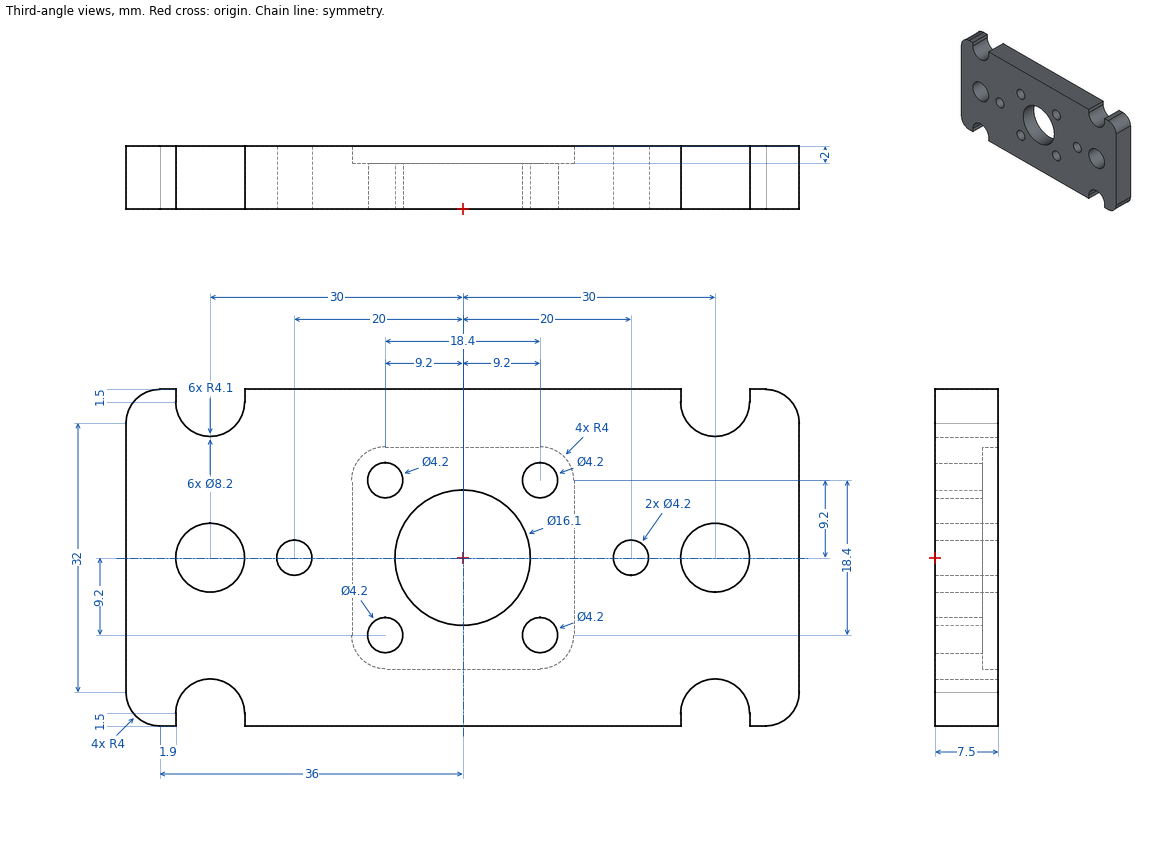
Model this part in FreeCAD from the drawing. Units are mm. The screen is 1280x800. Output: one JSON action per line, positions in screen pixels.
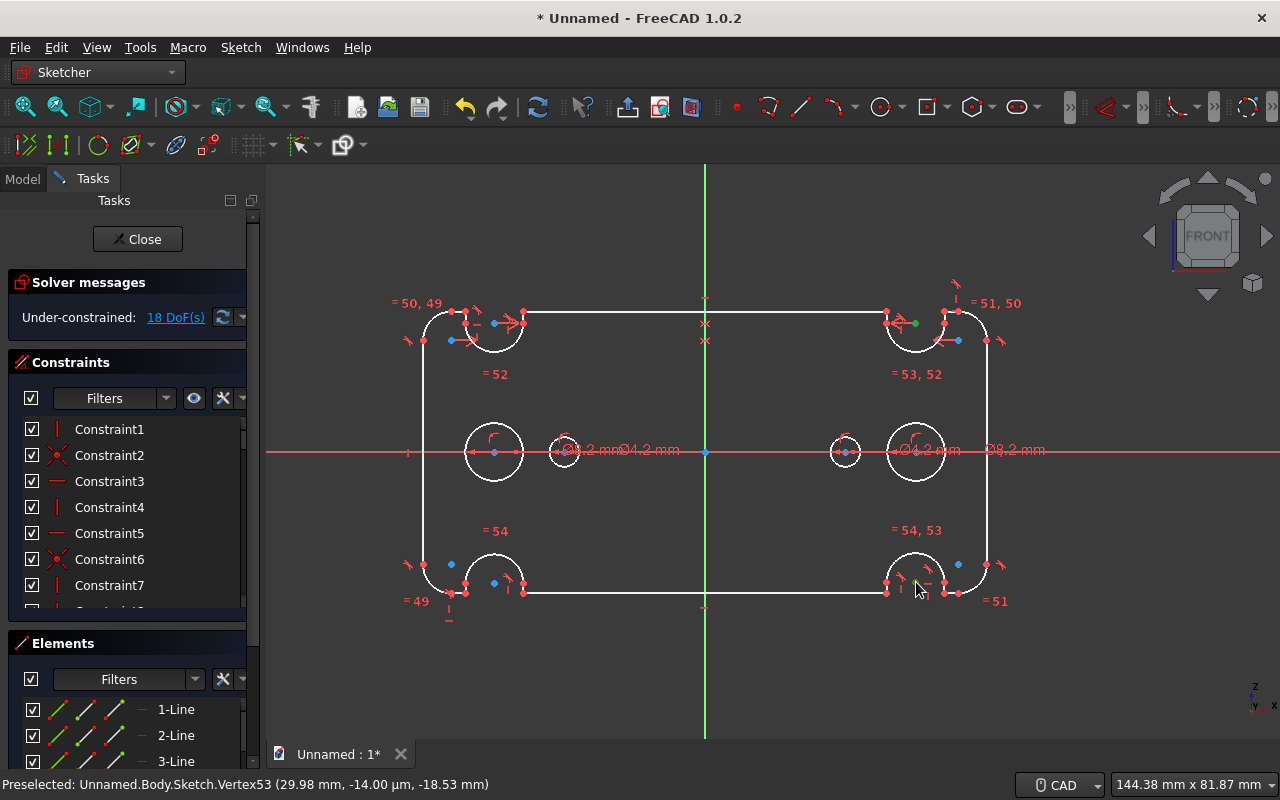
{"action": "left_click", "coordinate": [353, 452]}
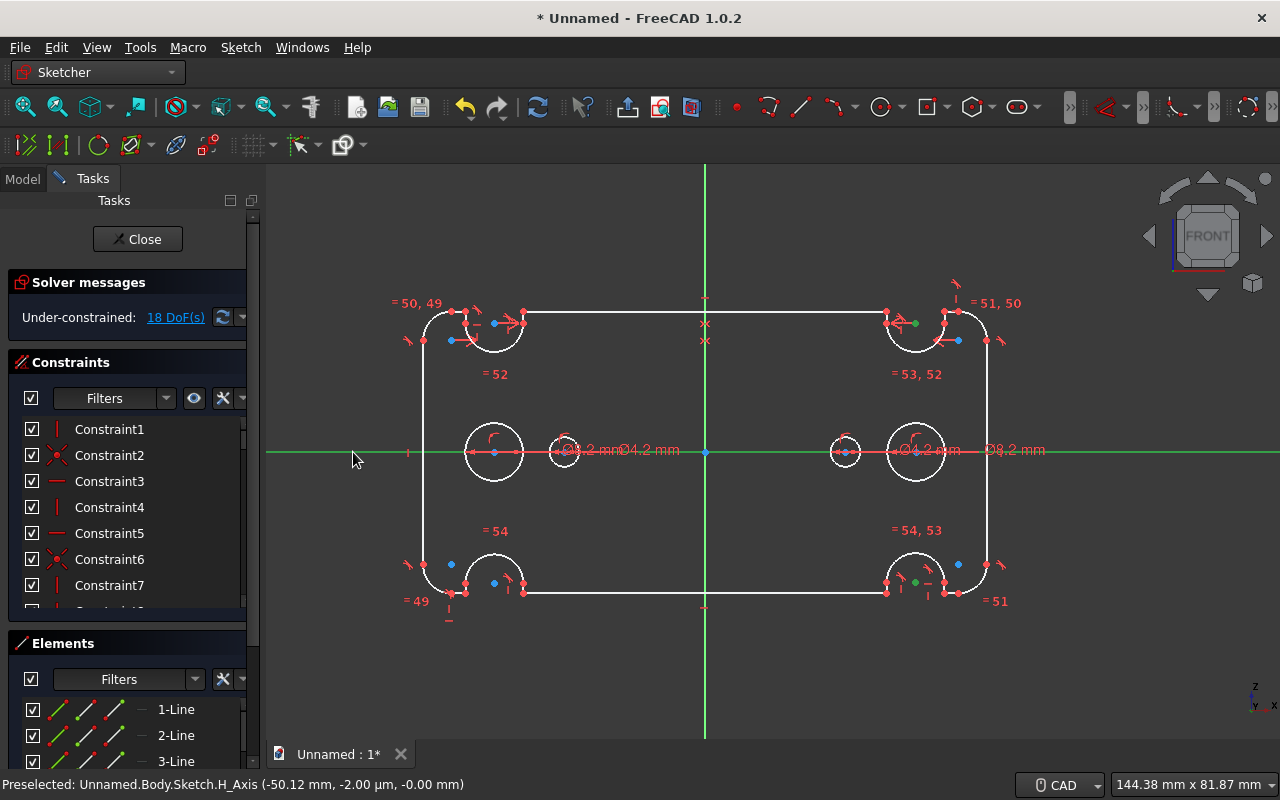
{"action": "key", "text": "s"}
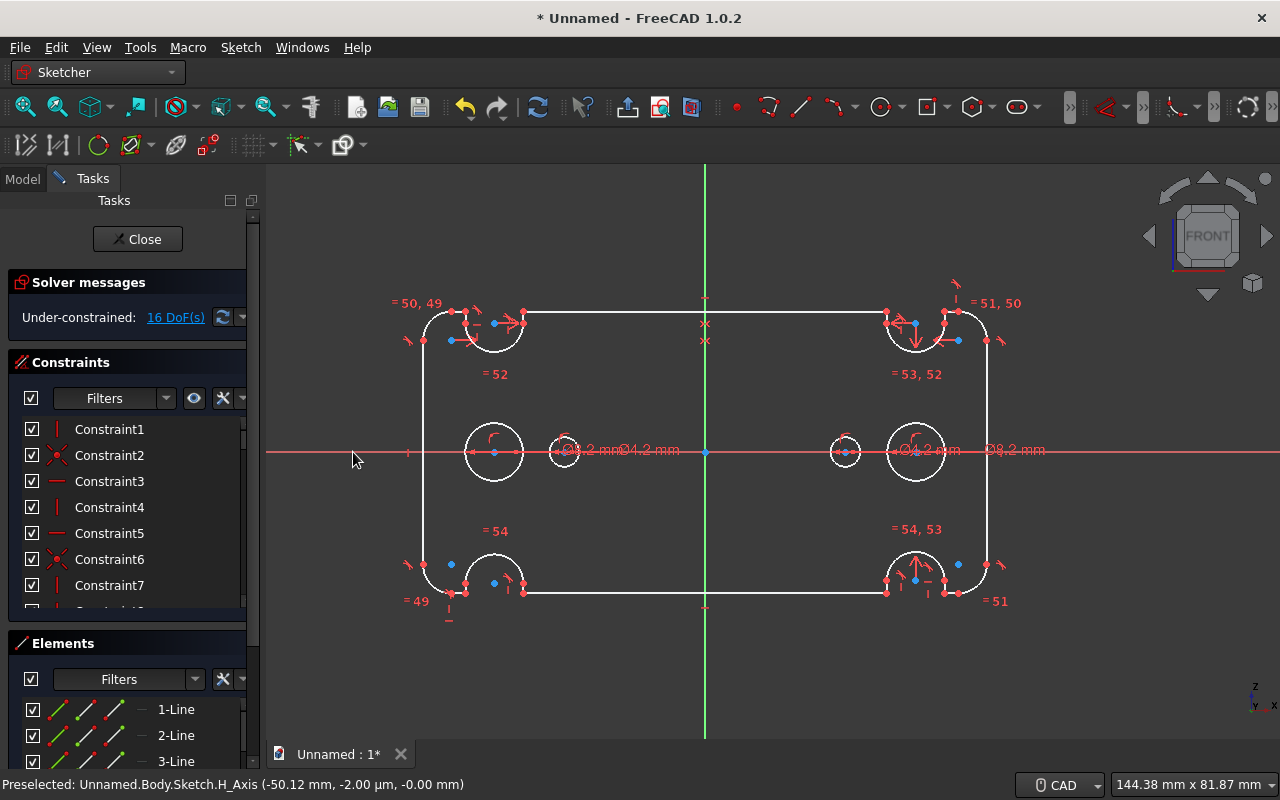
{"action": "left_click", "coordinate": [494, 323]}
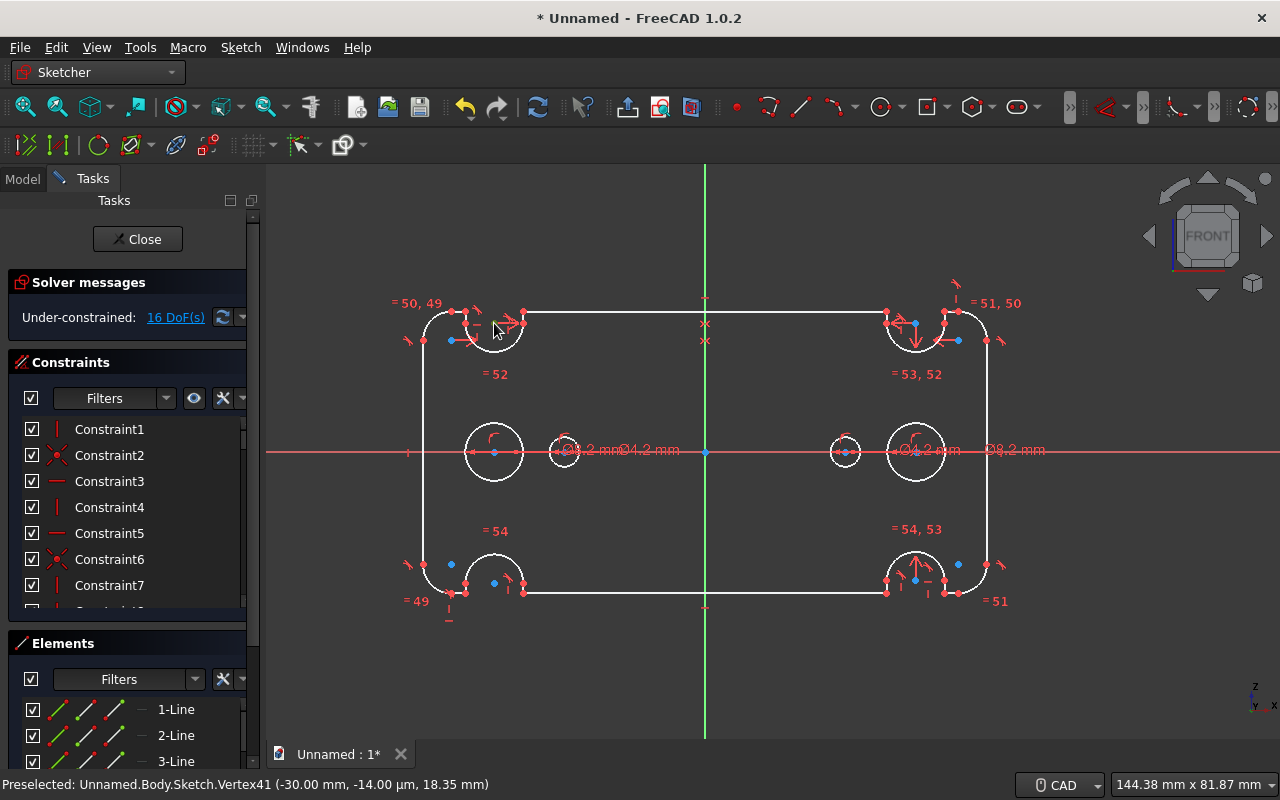
{"action": "left_click", "coordinate": [494, 583]}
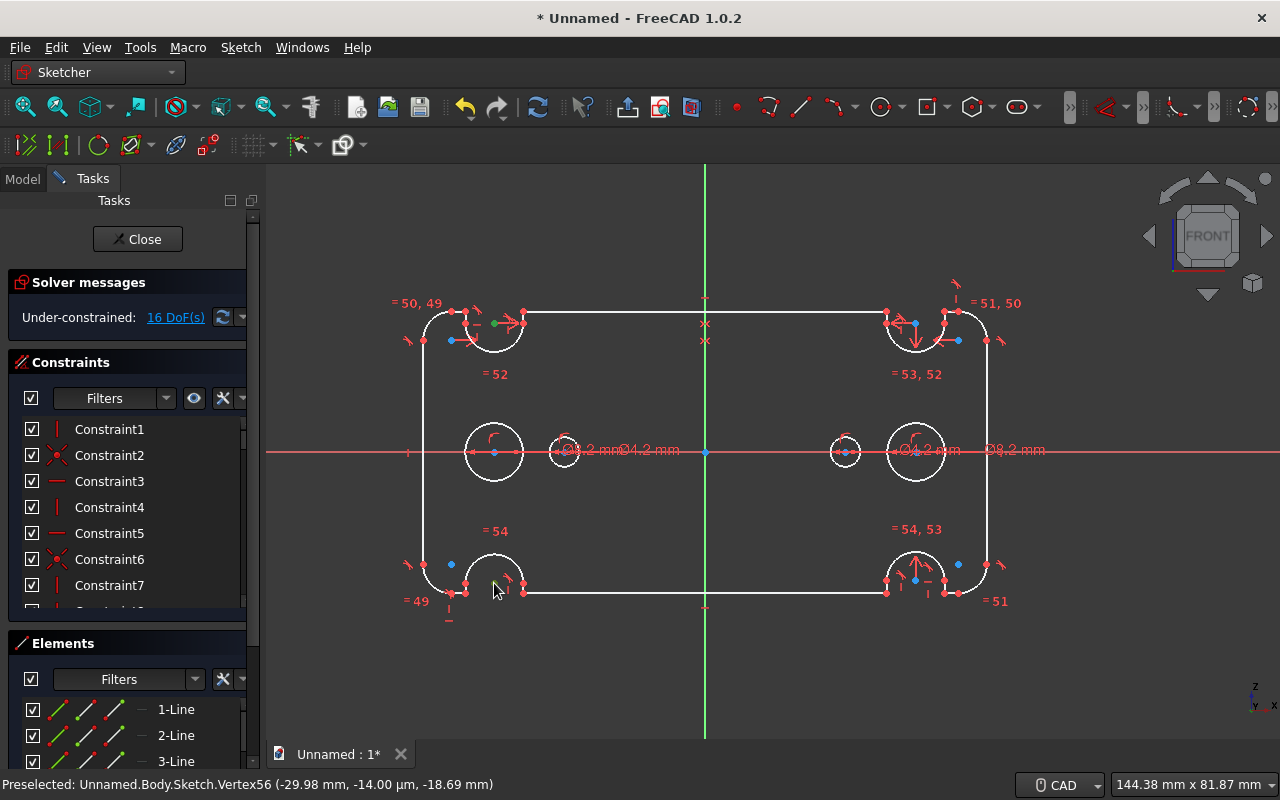
{"action": "left_click", "coordinate": [353, 452]}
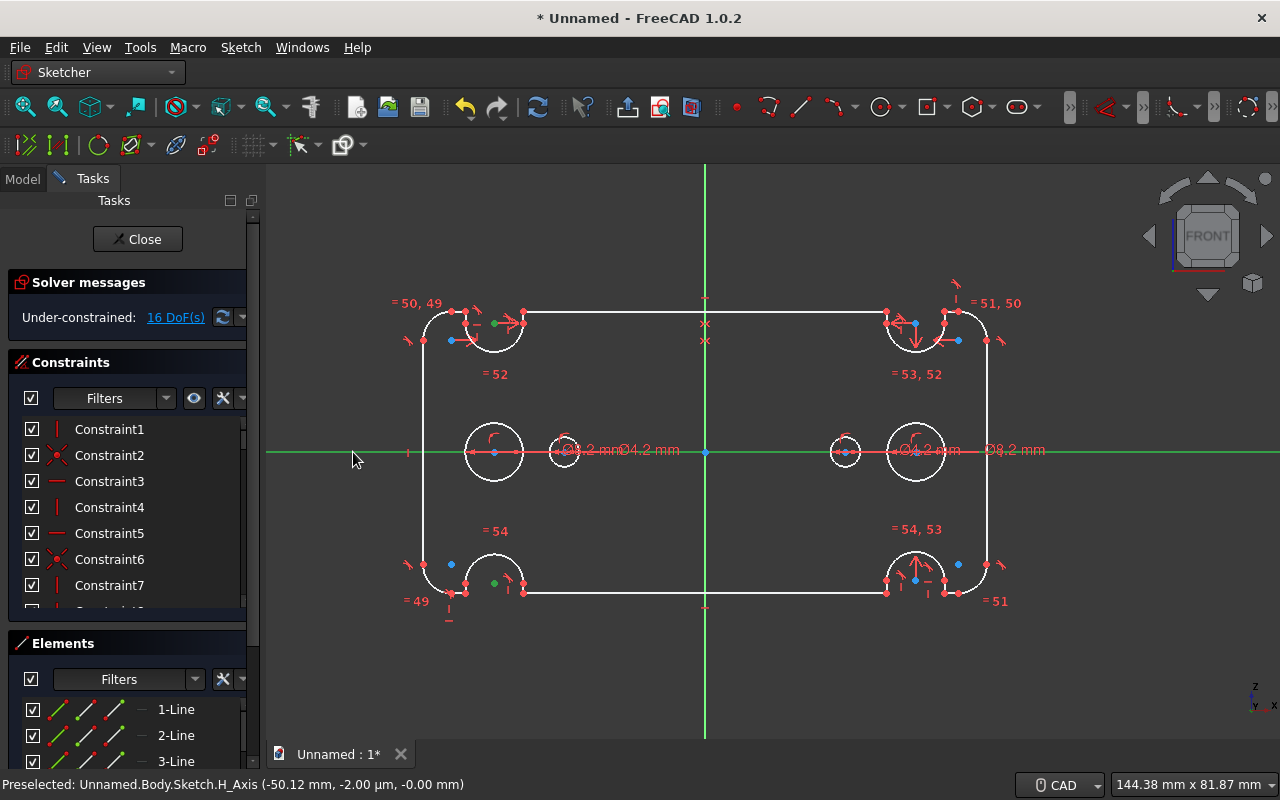
{"action": "key", "text": "s"}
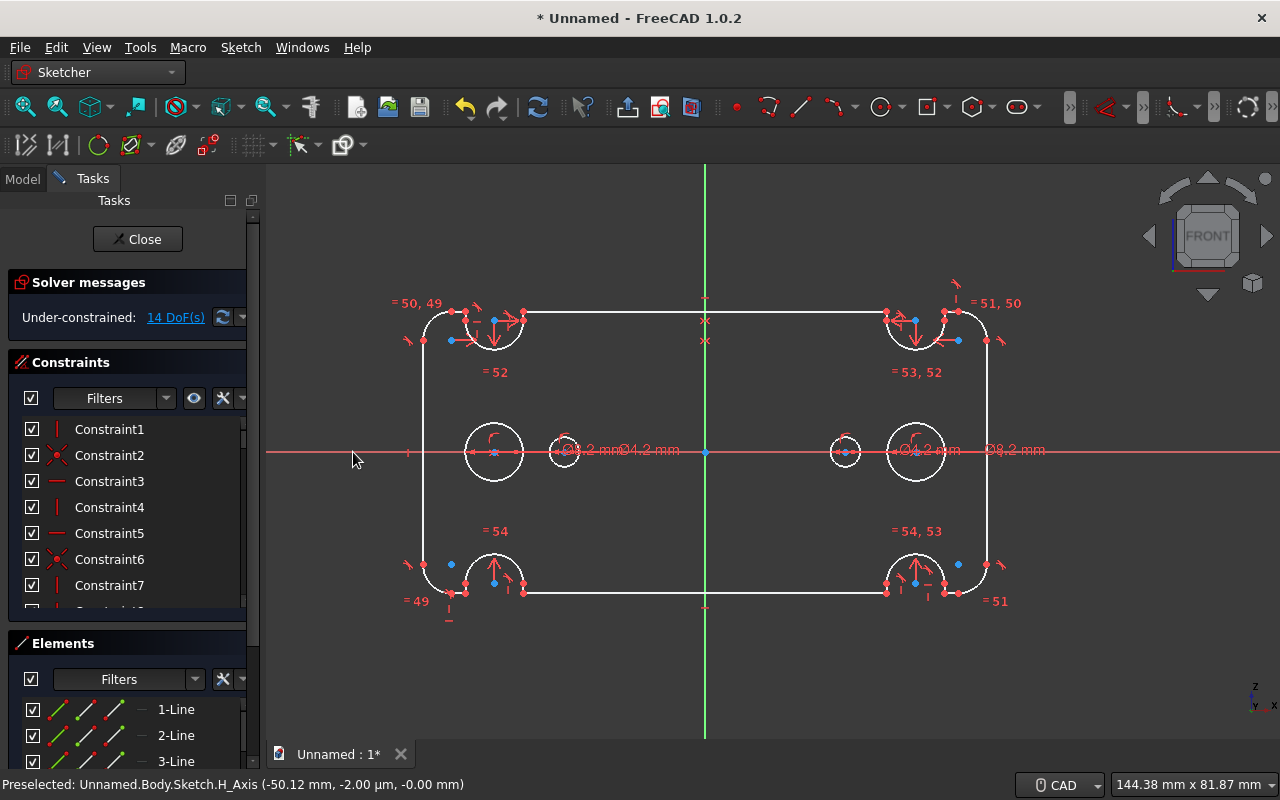
{"action": "left_click", "coordinate": [1106, 108]}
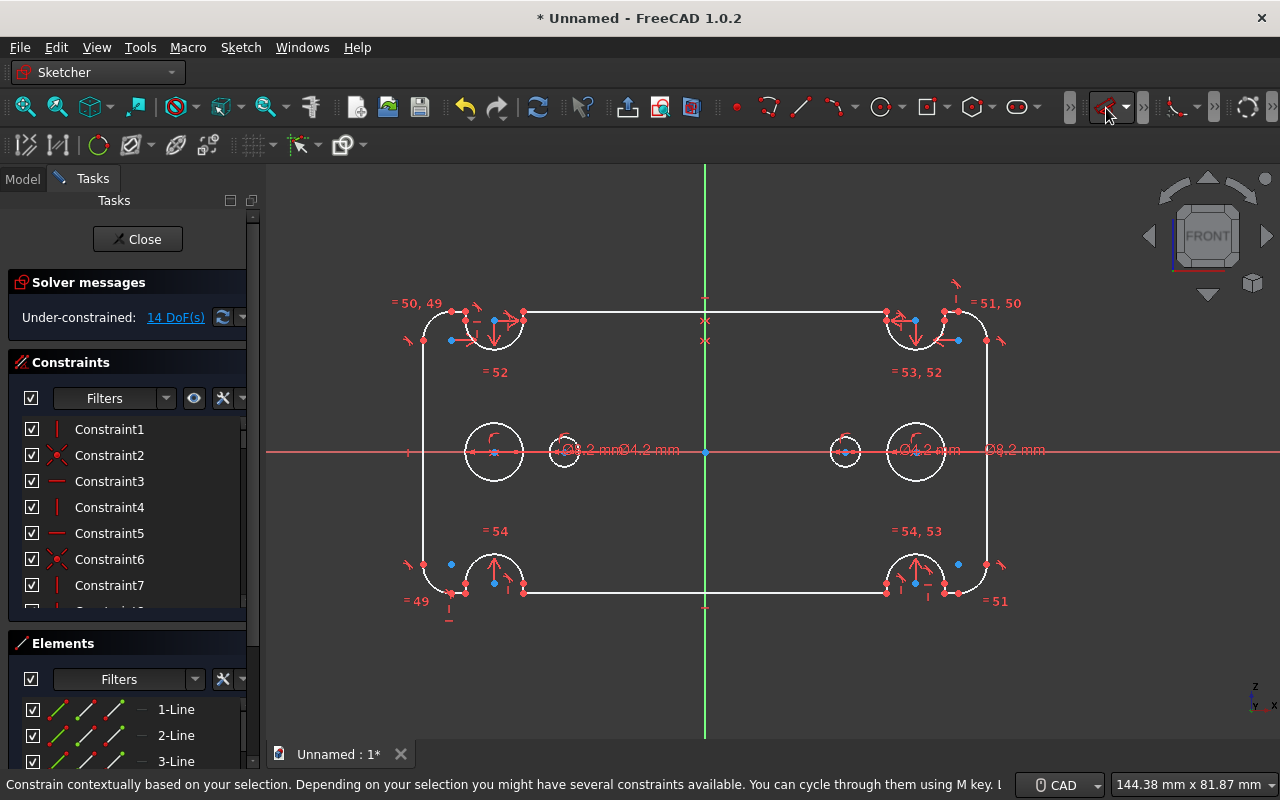
{"action": "scroll", "coordinate": [426, 578], "scroll_direction": "up", "scroll_amount": 2}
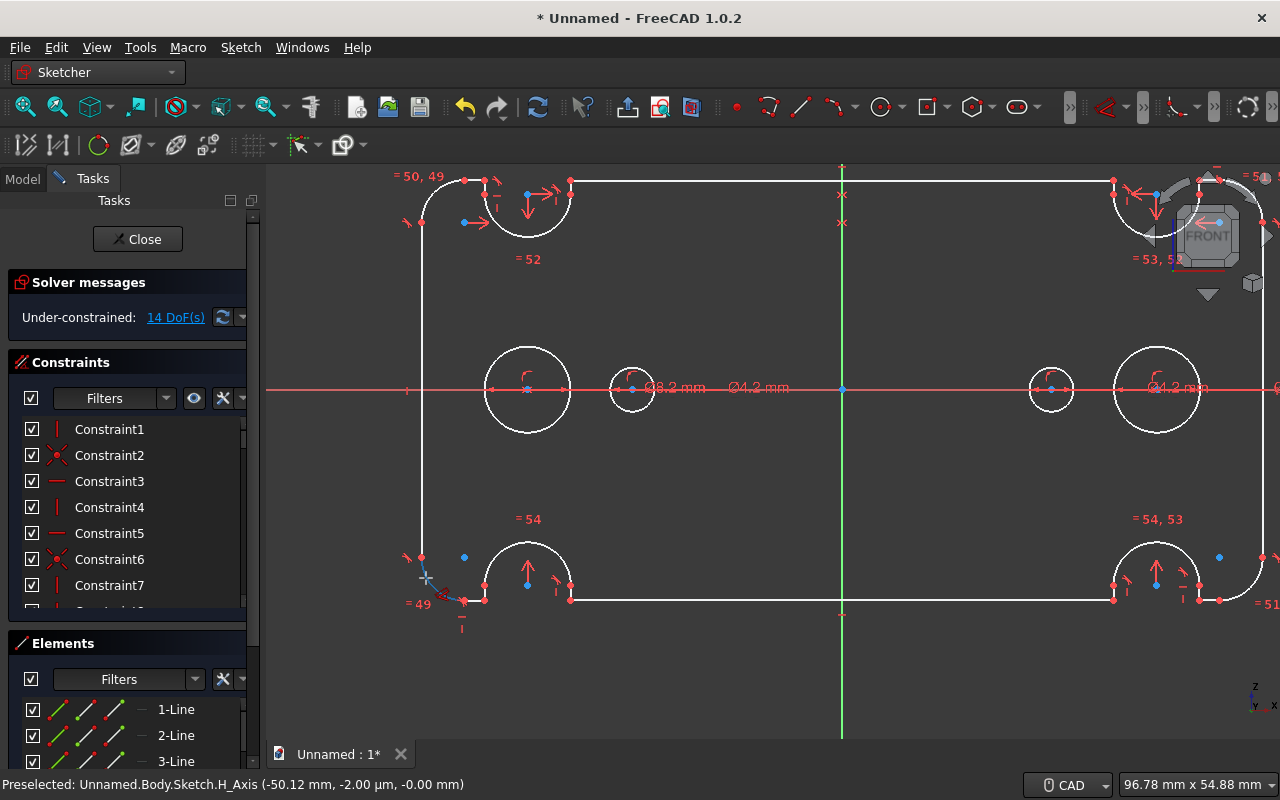
{"action": "left_click", "coordinate": [426, 577]}
{"action": "left_click", "coordinate": [397, 591]}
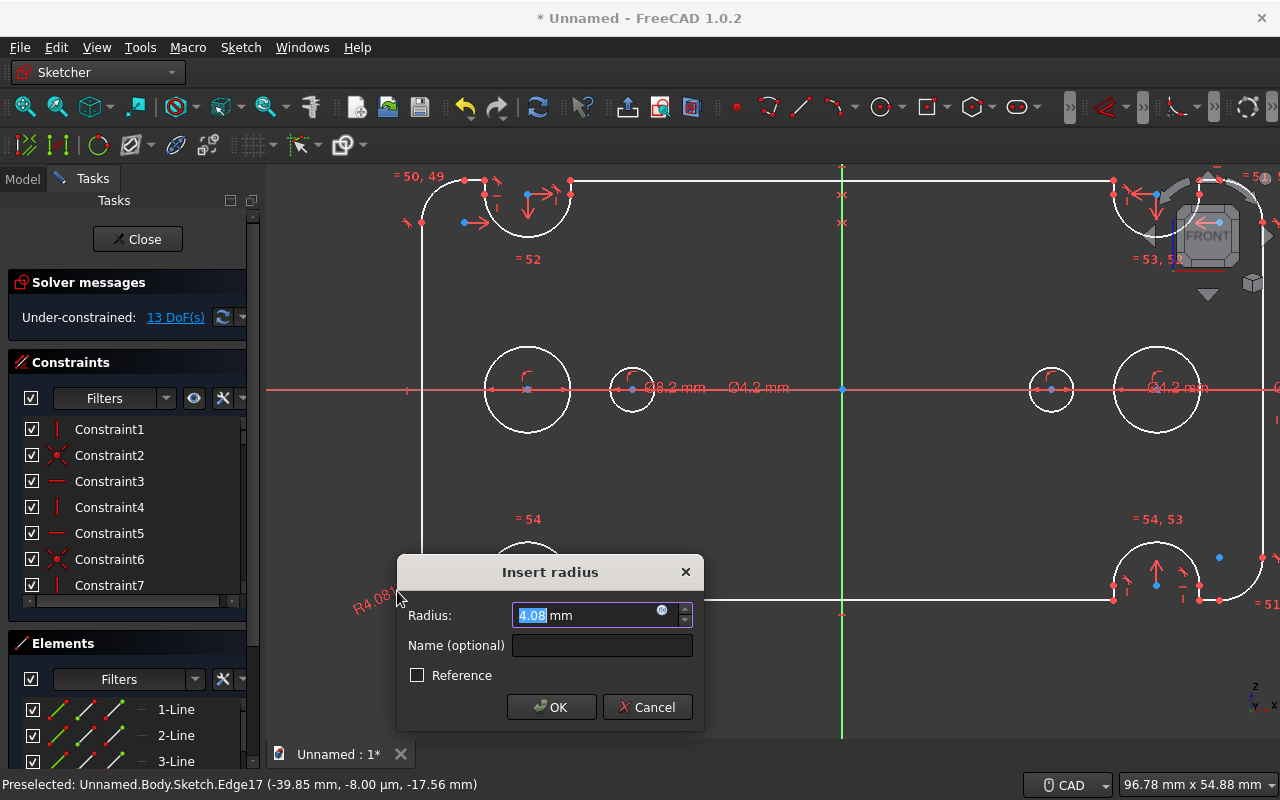
{"action": "type", "text": "4"}
{"action": "key", "text": "Return"}